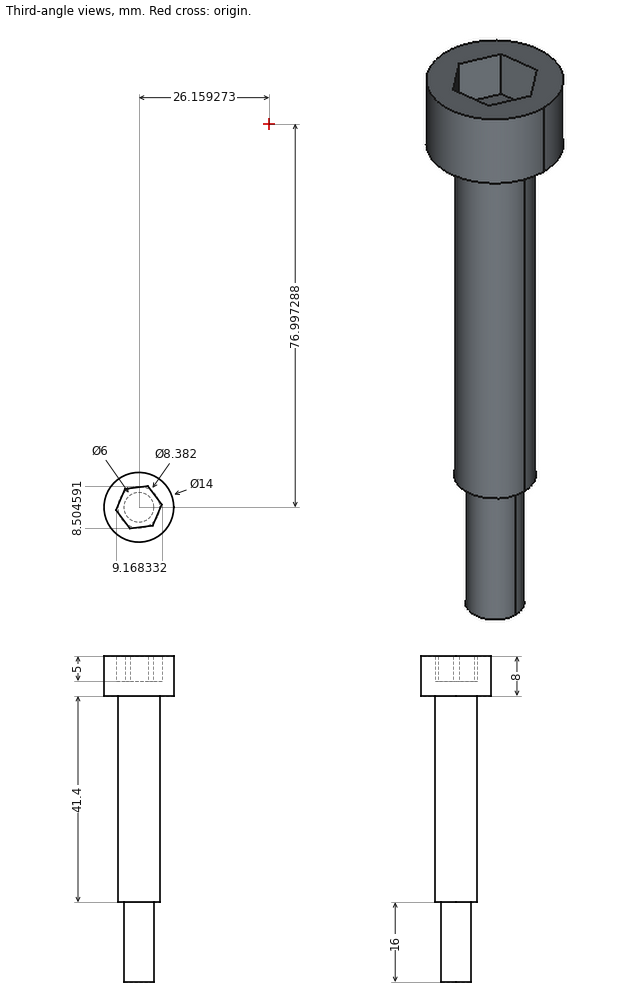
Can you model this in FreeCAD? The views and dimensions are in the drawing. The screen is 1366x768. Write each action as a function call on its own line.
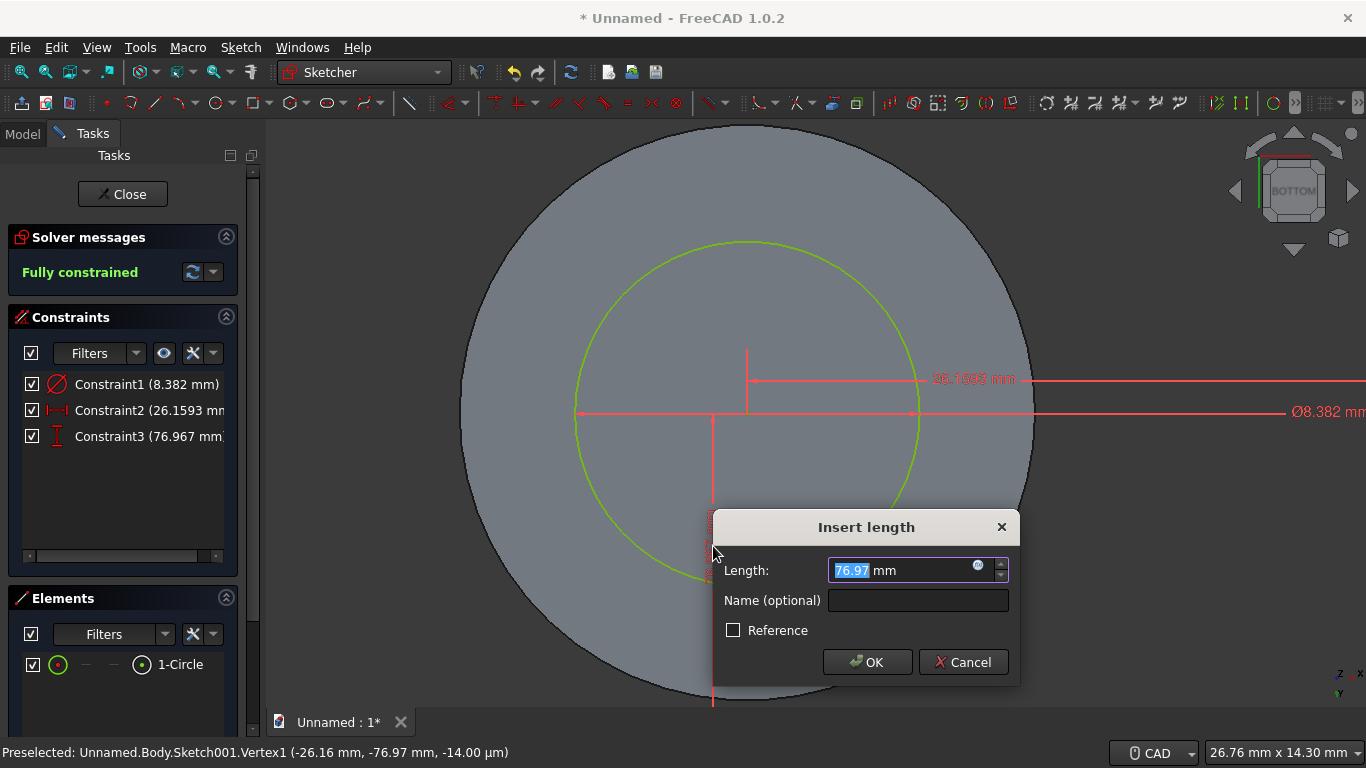
text(76.997288)
key(Return)
key(Escape)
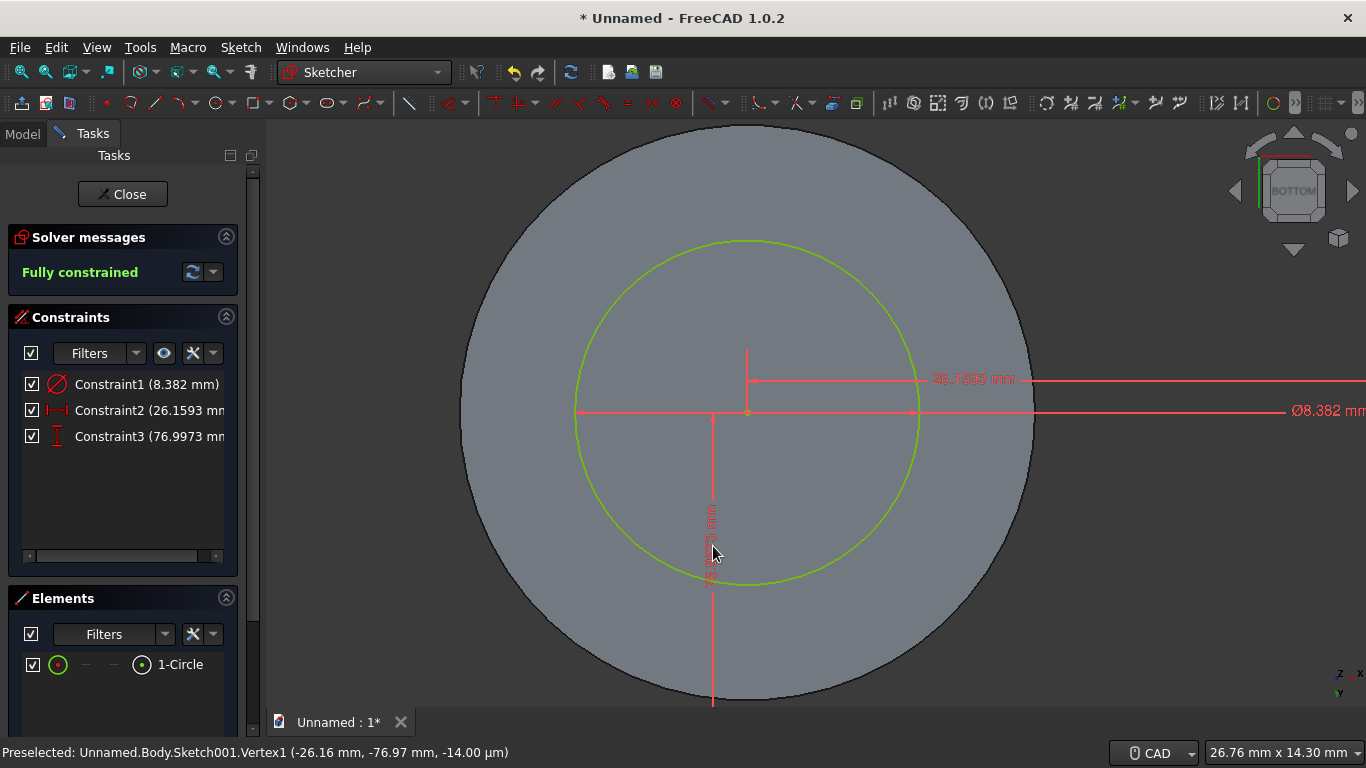
click(123, 194)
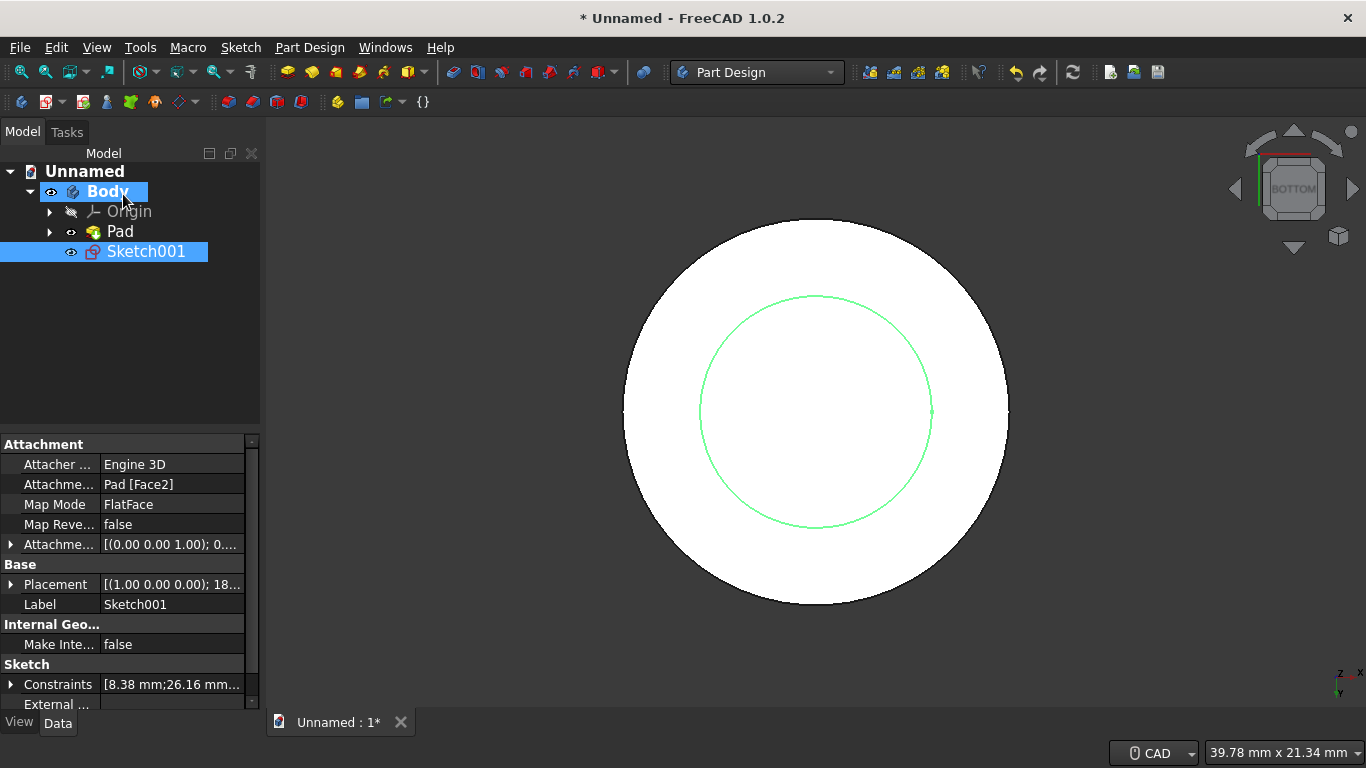
click(288, 72)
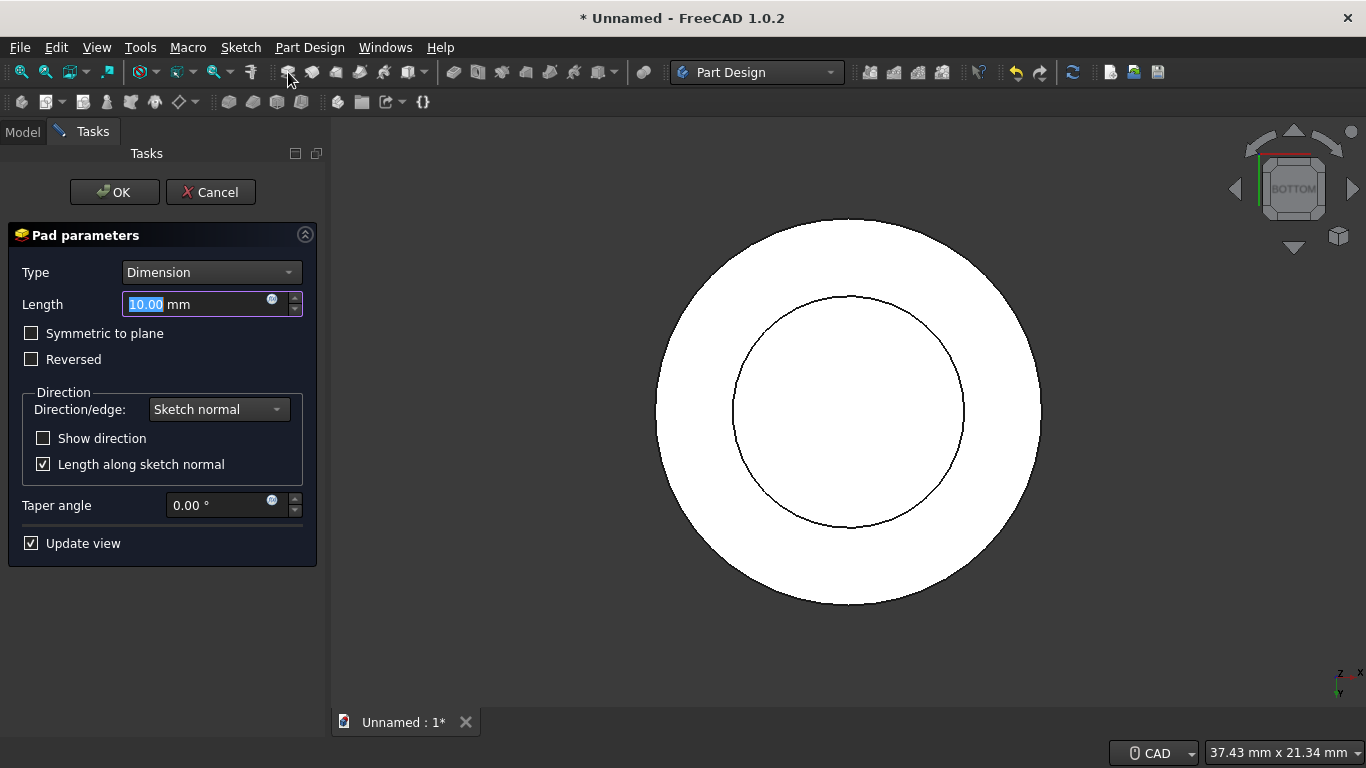
text(41.4)
key(Tab)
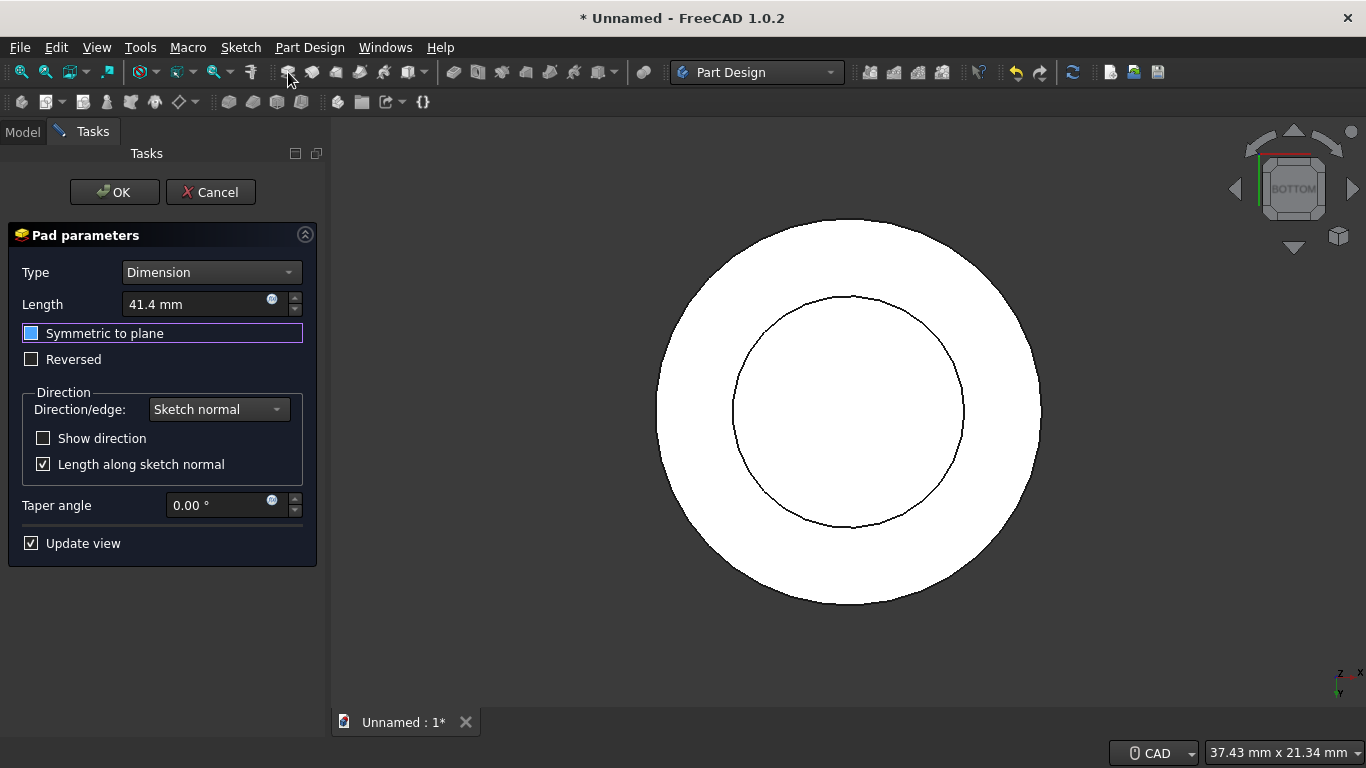
click(115, 192)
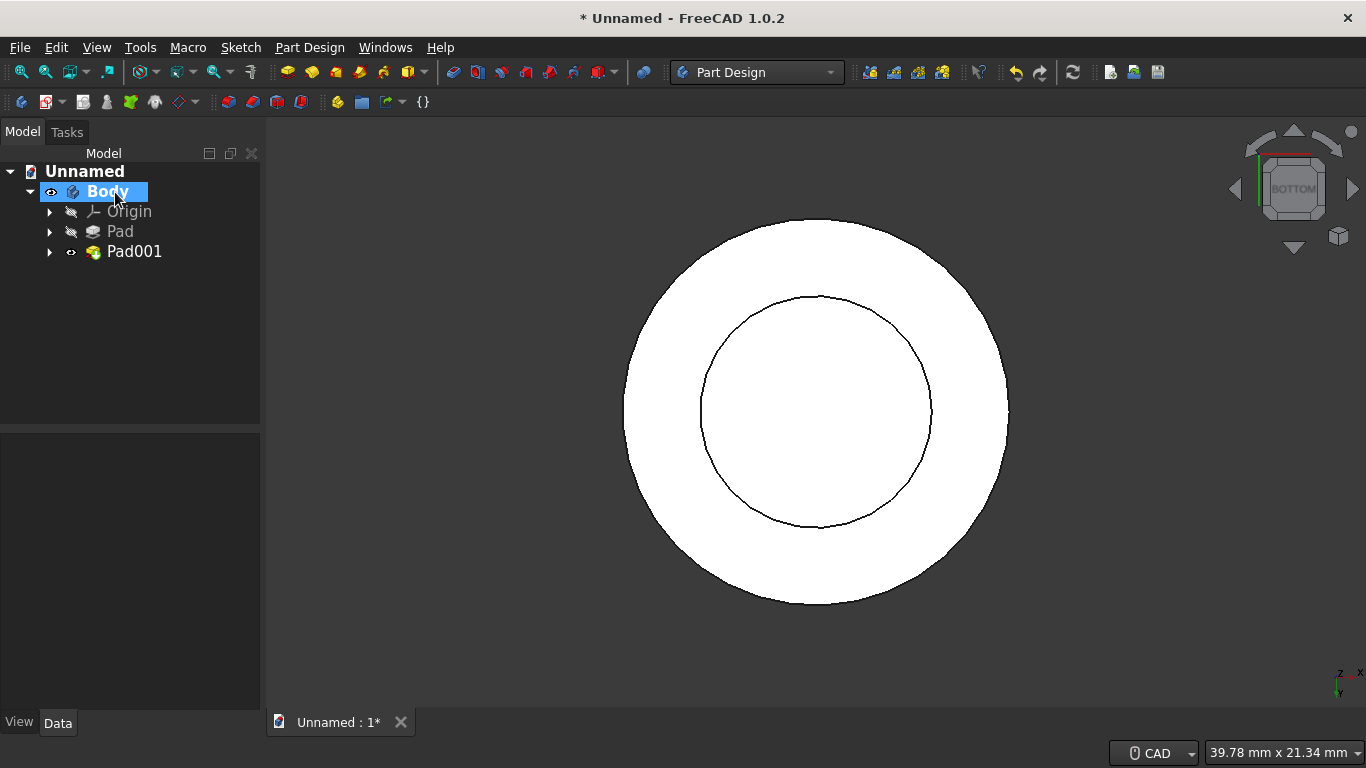
click(816, 411)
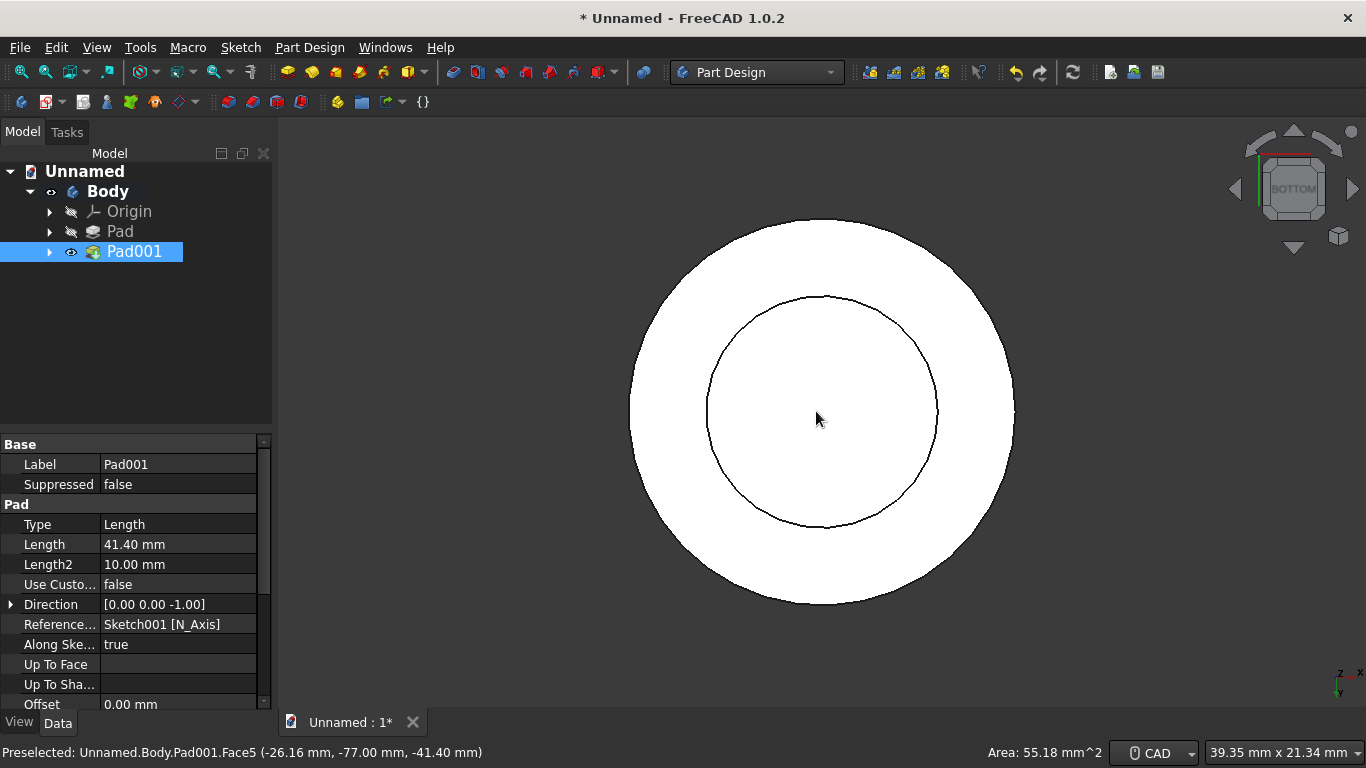
click(46, 102)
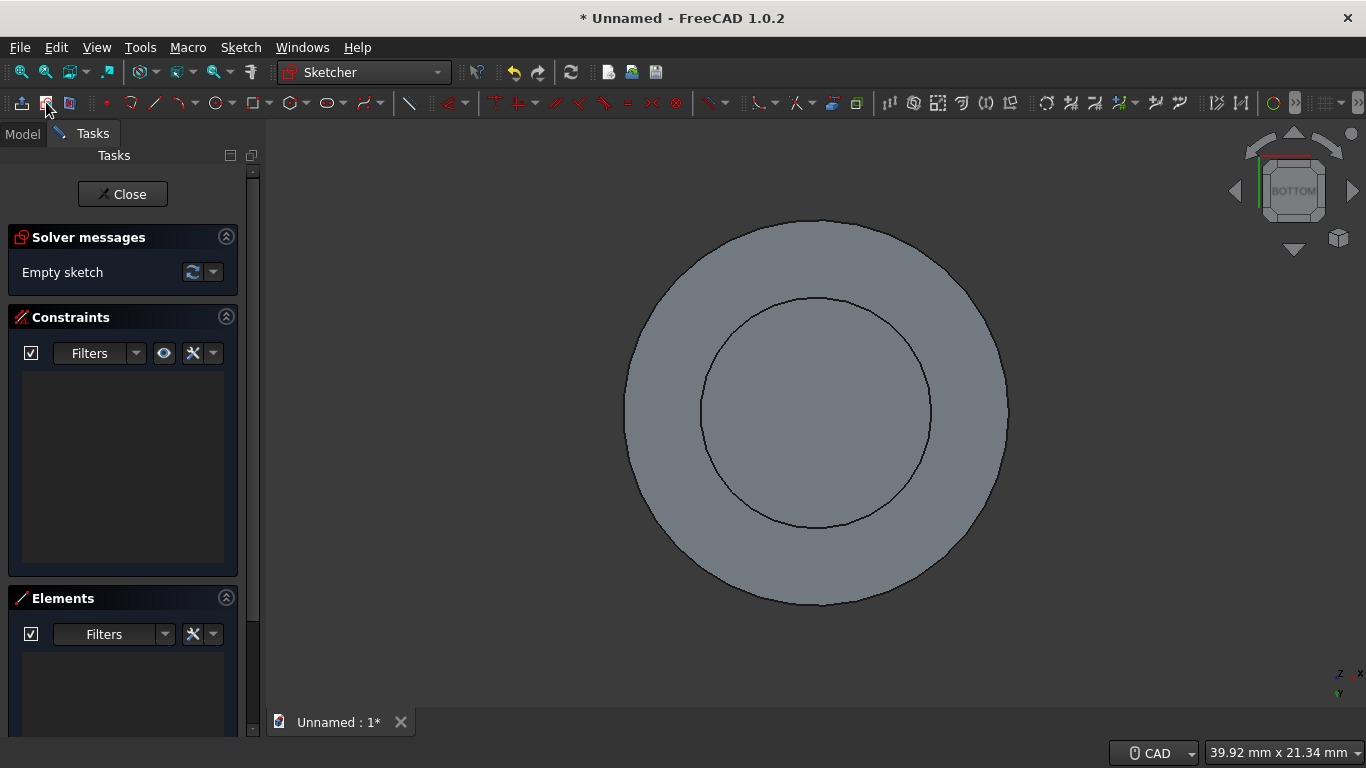
scroll(872, 413, up, 4)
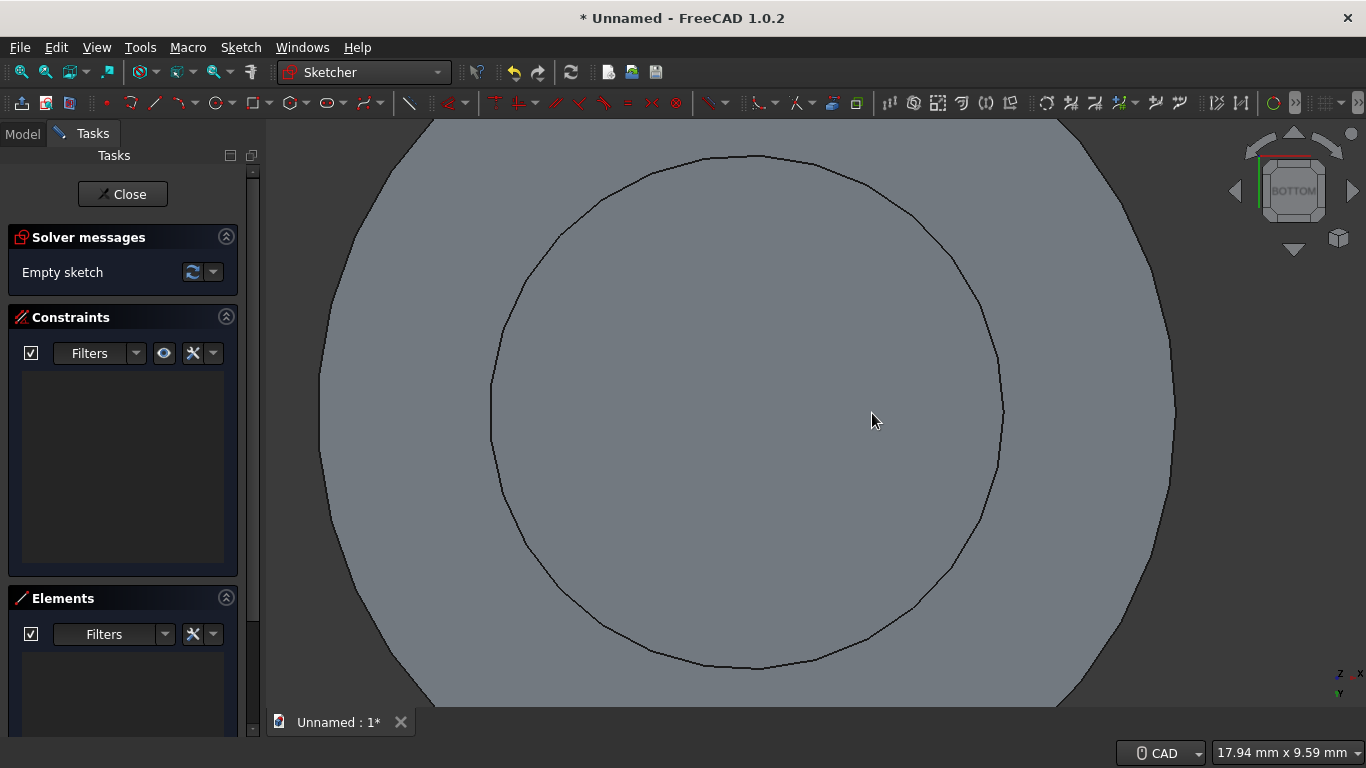
key(g)
key(c)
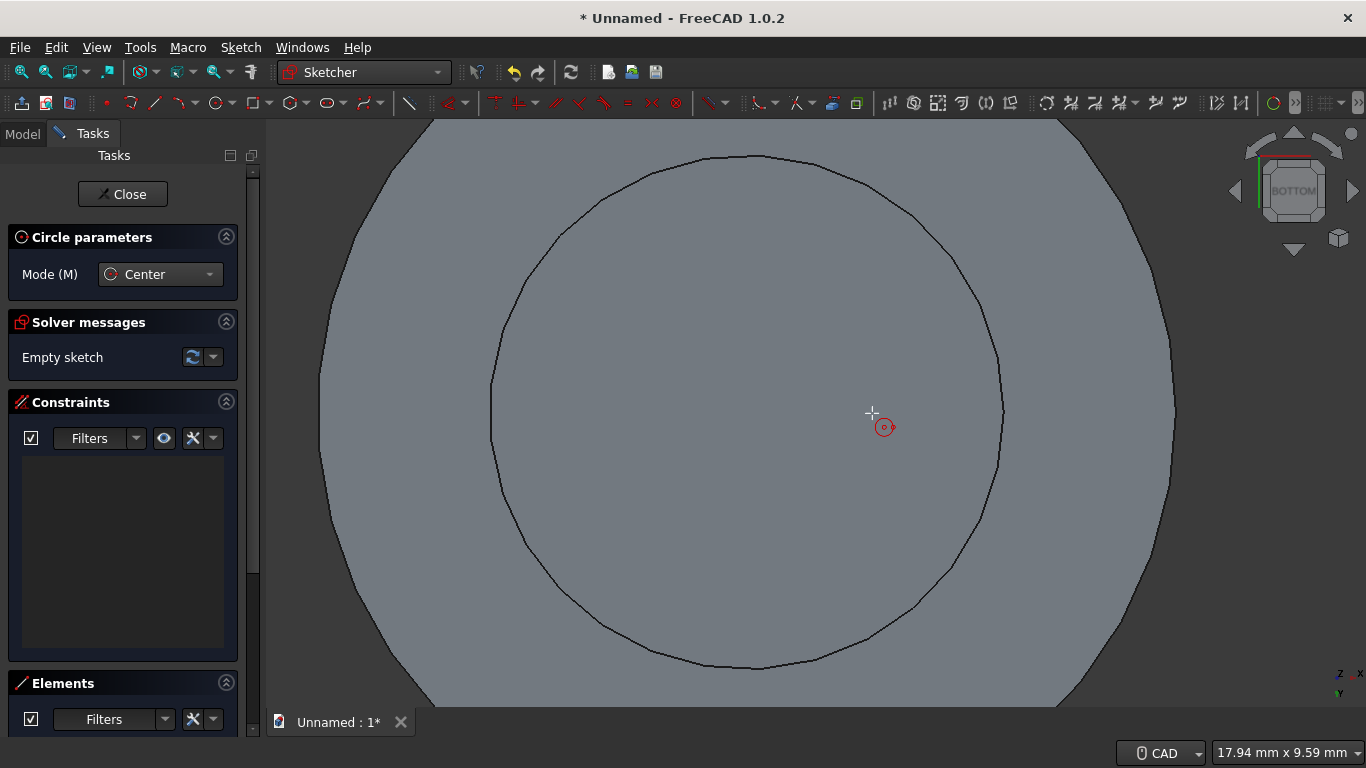
click(747, 412)
move(877, 282)